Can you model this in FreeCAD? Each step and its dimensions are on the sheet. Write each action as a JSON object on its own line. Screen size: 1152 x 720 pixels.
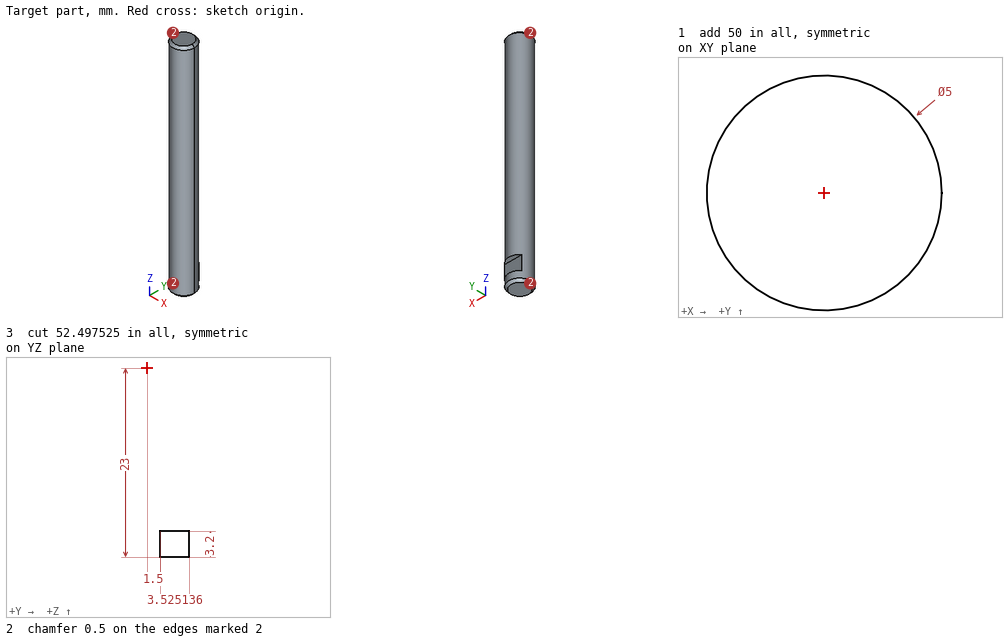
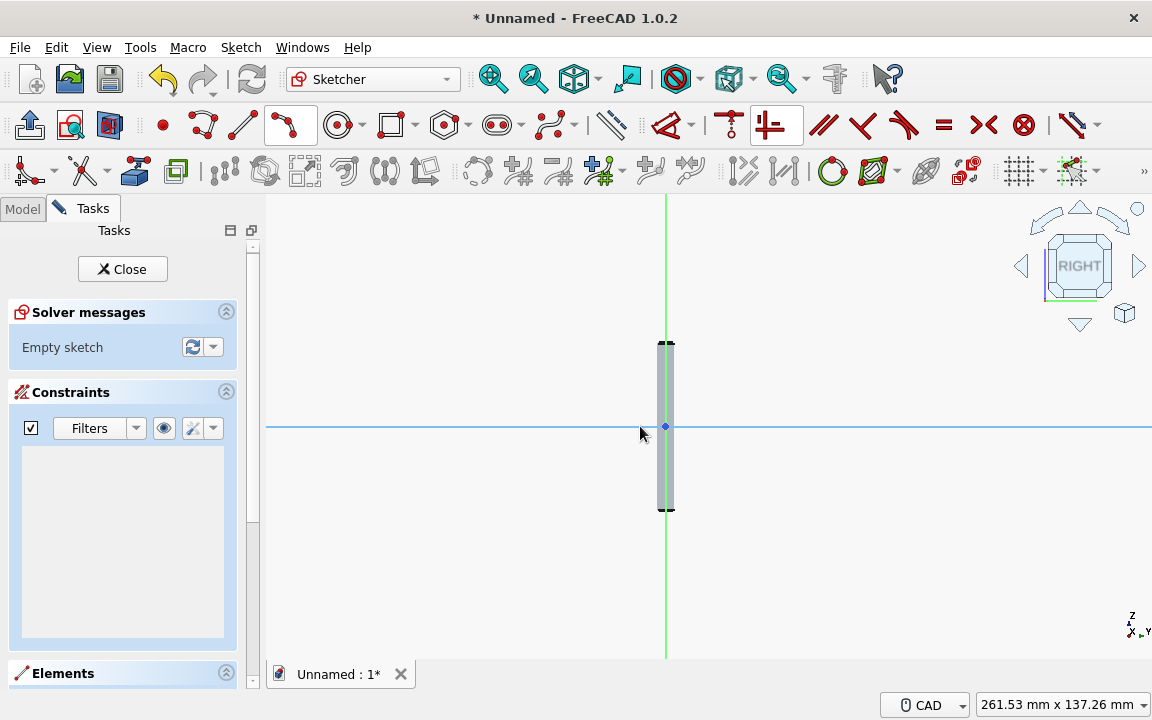
{"action": "scroll", "coordinate": [679, 503], "scroll_direction": "up", "scroll_amount": 15}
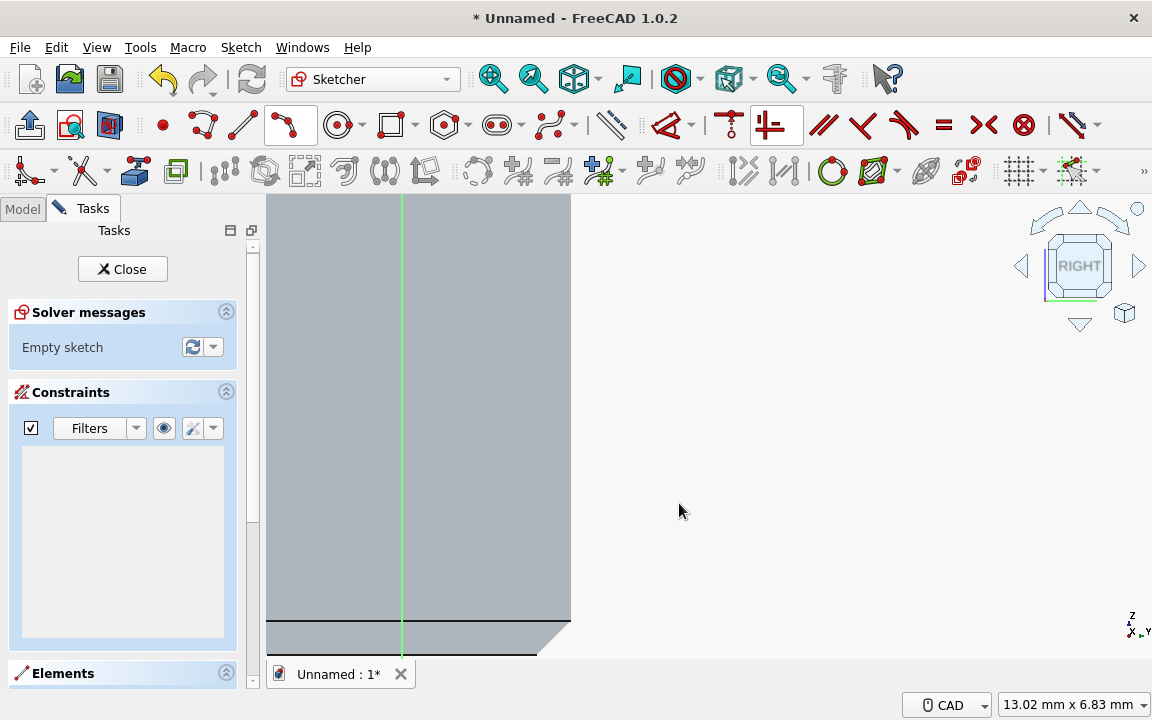
{"action": "key", "text": "g r"}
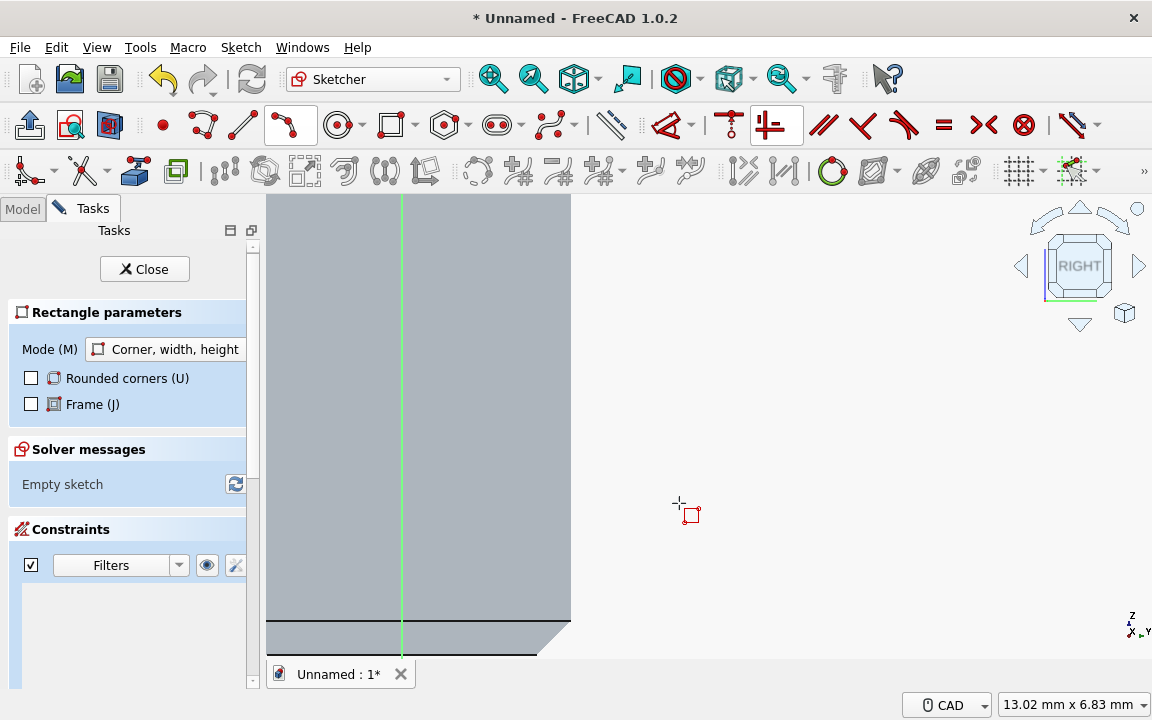
{"action": "left_click", "coordinate": [504, 301]}
{"action": "mouse_move", "coordinate": [744, 519]}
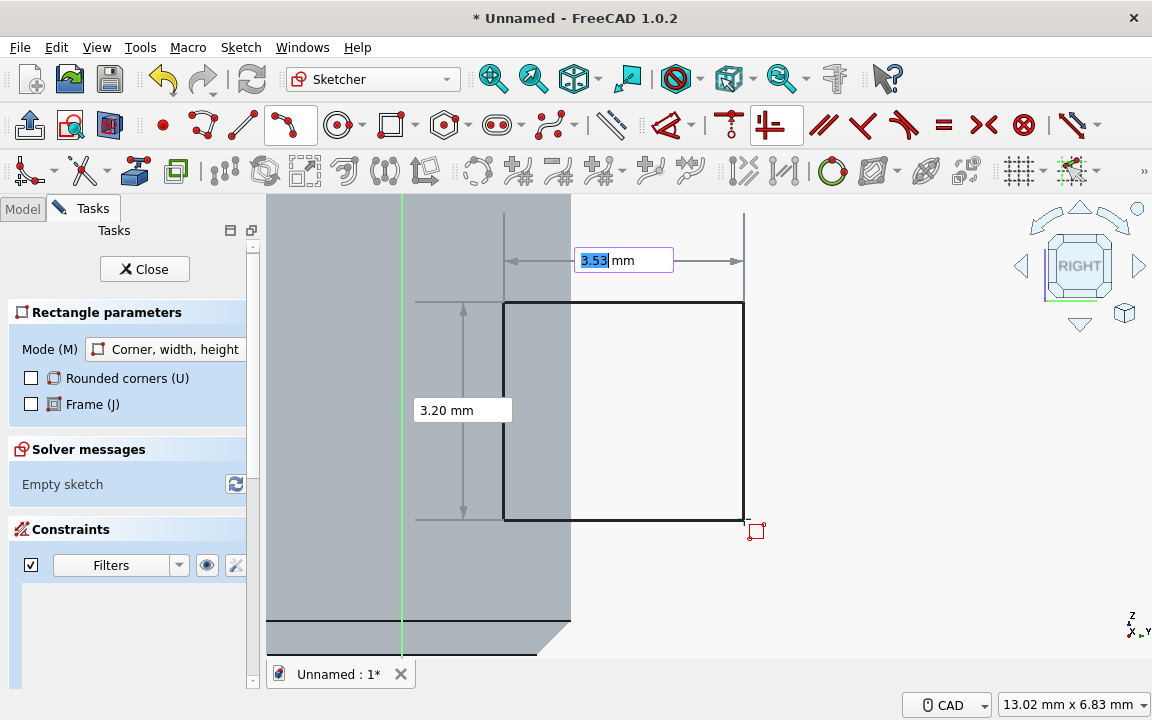
{"action": "type", "text": "3.525136"}
{"action": "key", "text": "Tab"}
{"action": "type", "text": "3.2"}
{"action": "key", "text": "Return"}
{"action": "key", "text": "Escape"}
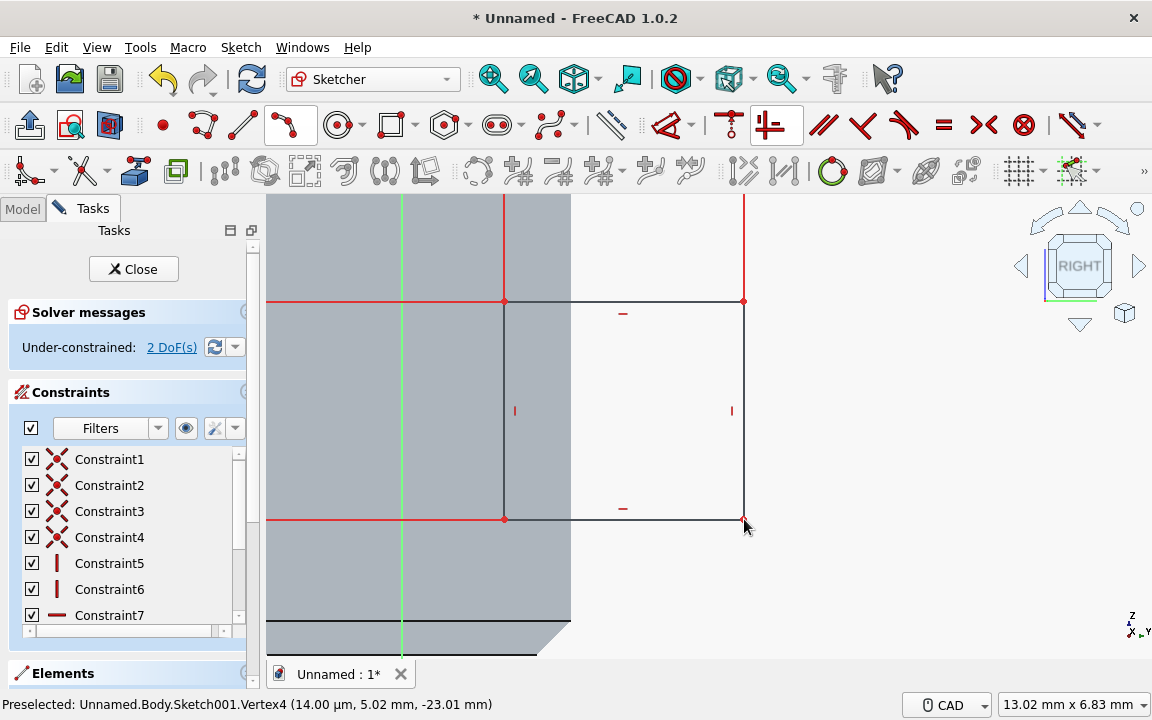
{"action": "left_click", "coordinate": [504, 520]}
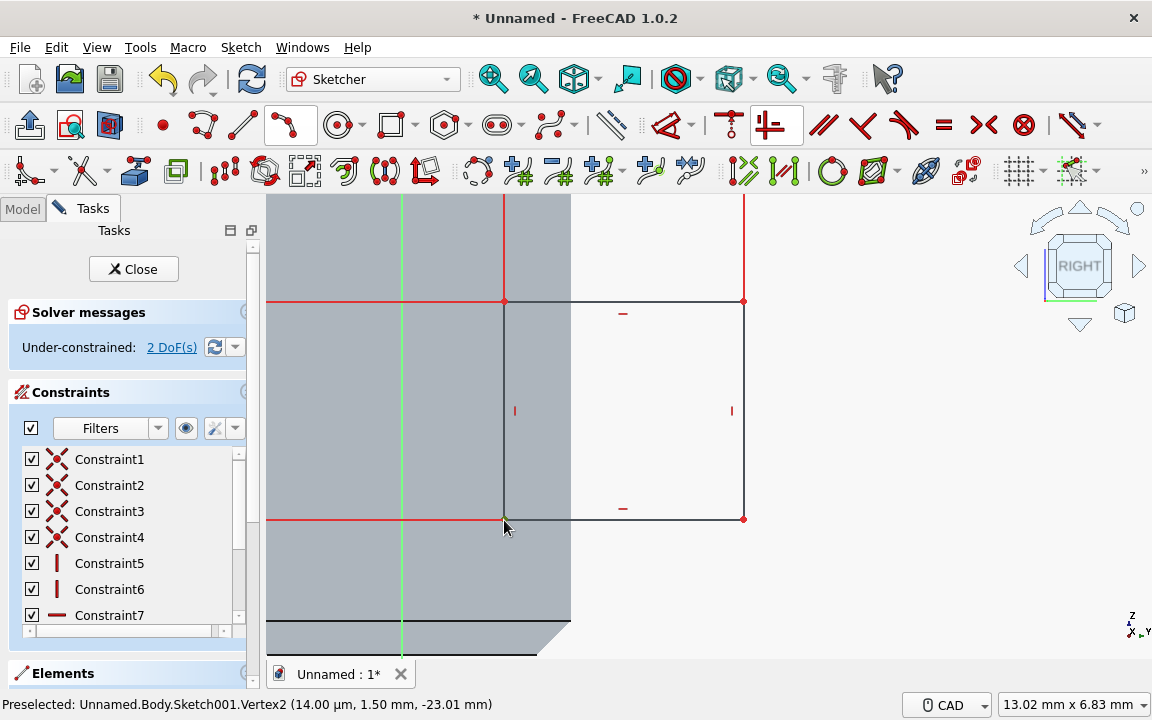
{"action": "key", "text": "i"}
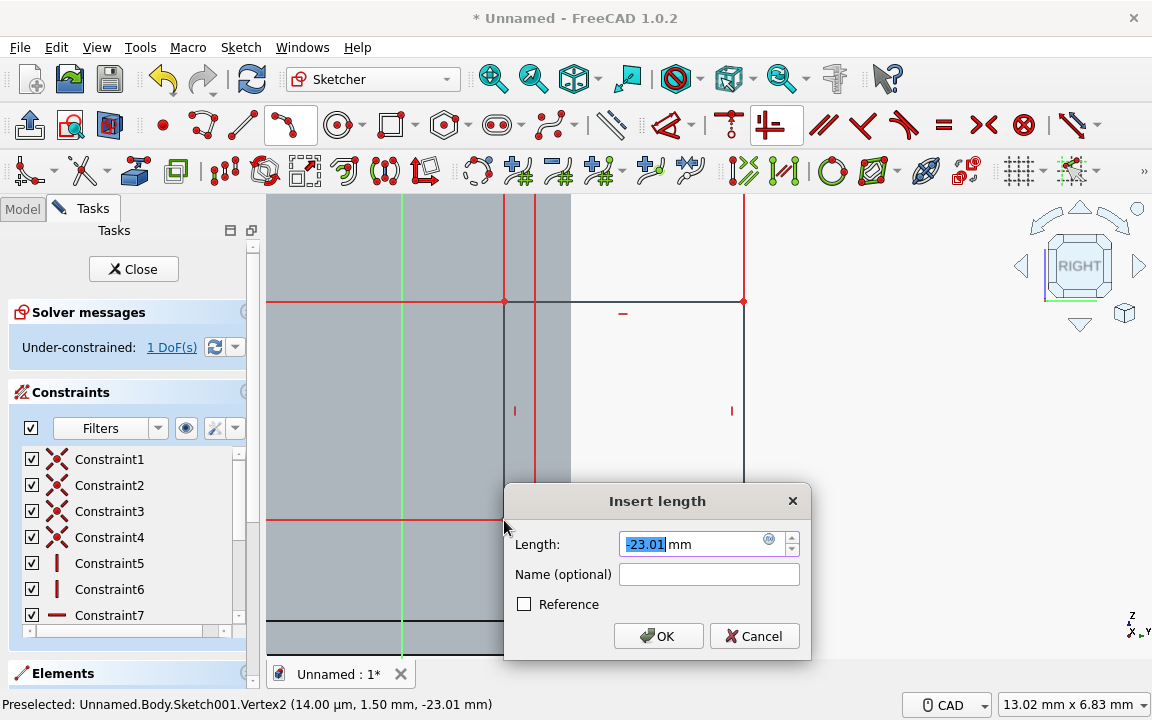
{"action": "type", "text": "-23"}
{"action": "key", "text": "Return"}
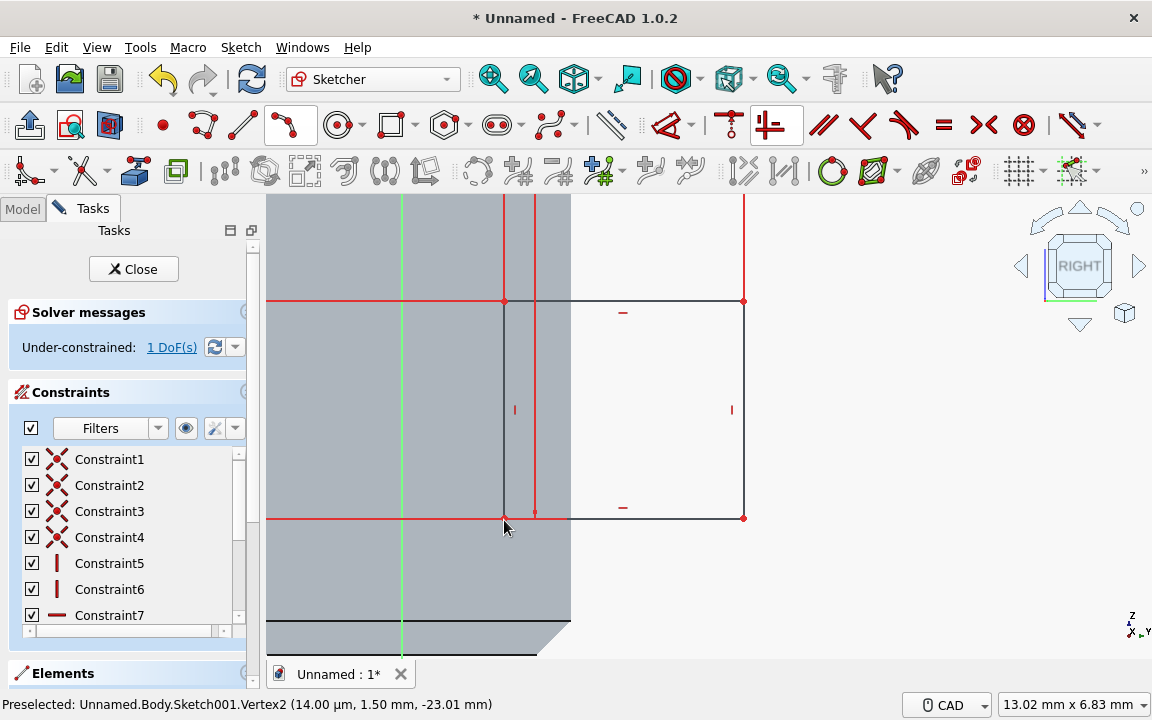
{"action": "left_click", "coordinate": [504, 301]}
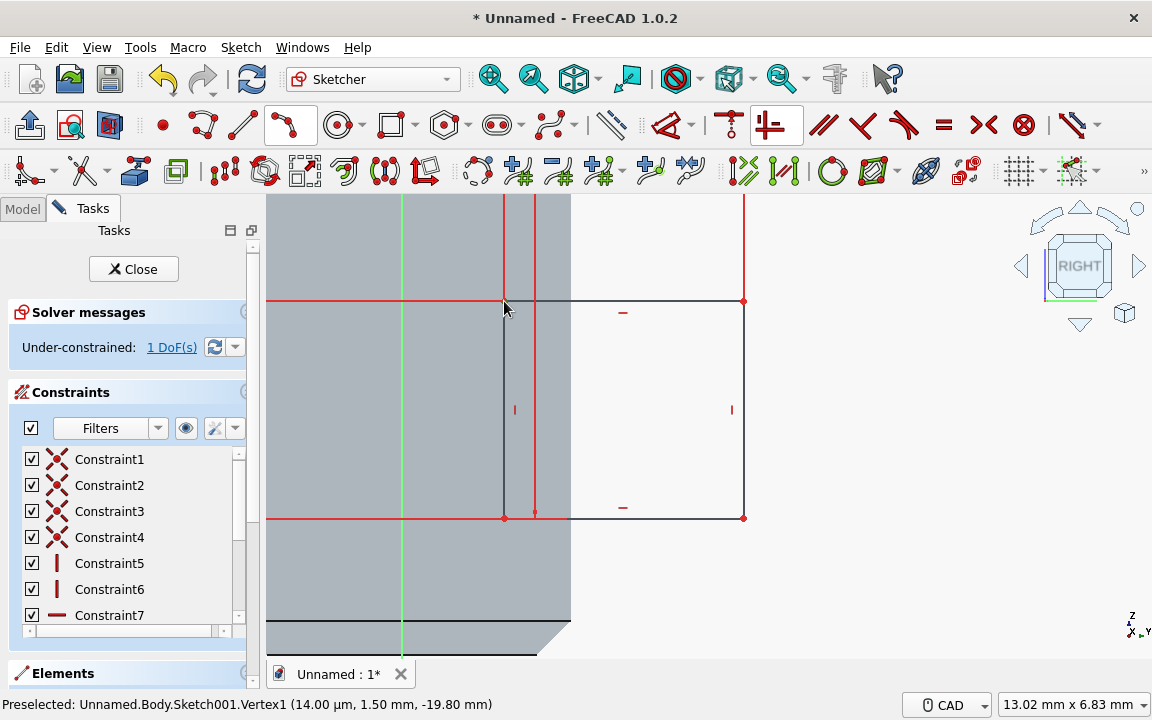
{"action": "key", "text": "l"}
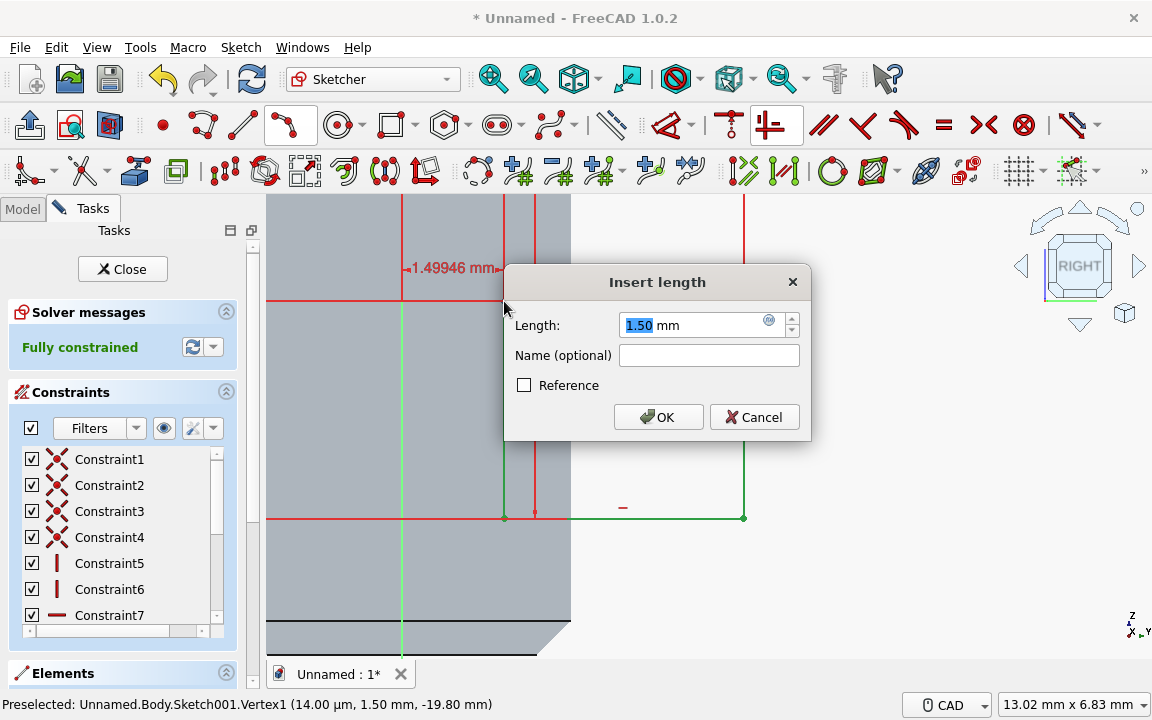
{"action": "type", "text": "1.5"}
{"action": "key", "text": "Return"}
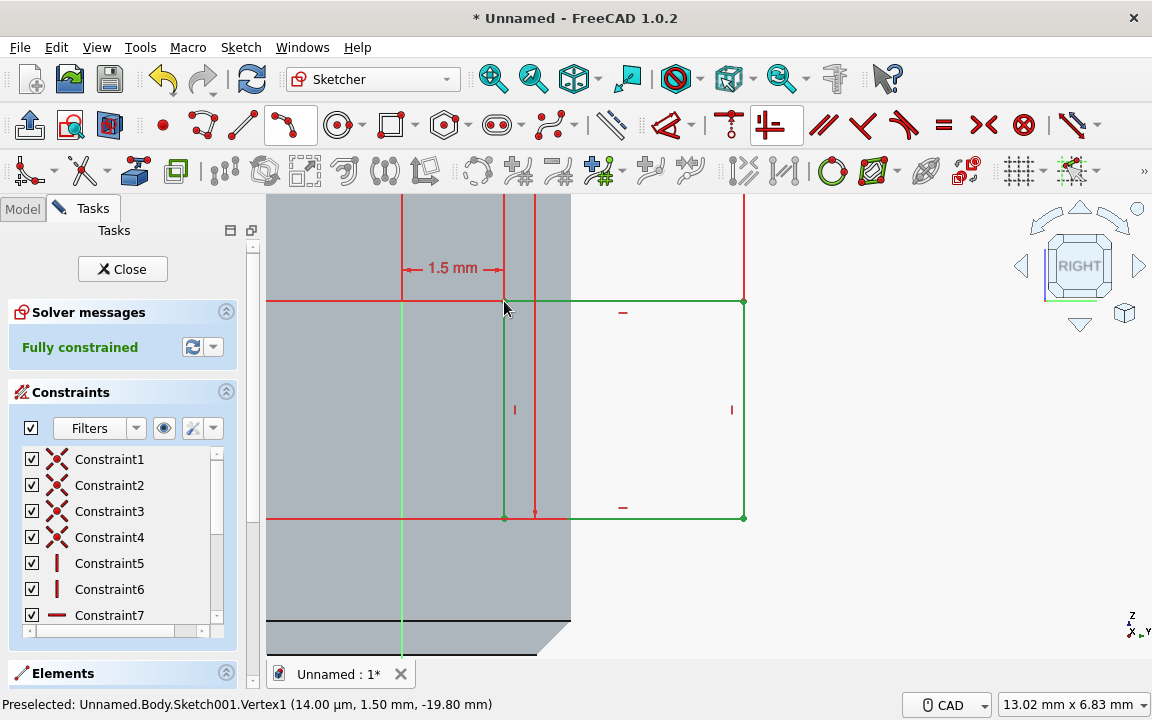
{"action": "left_click", "coordinate": [123, 269]}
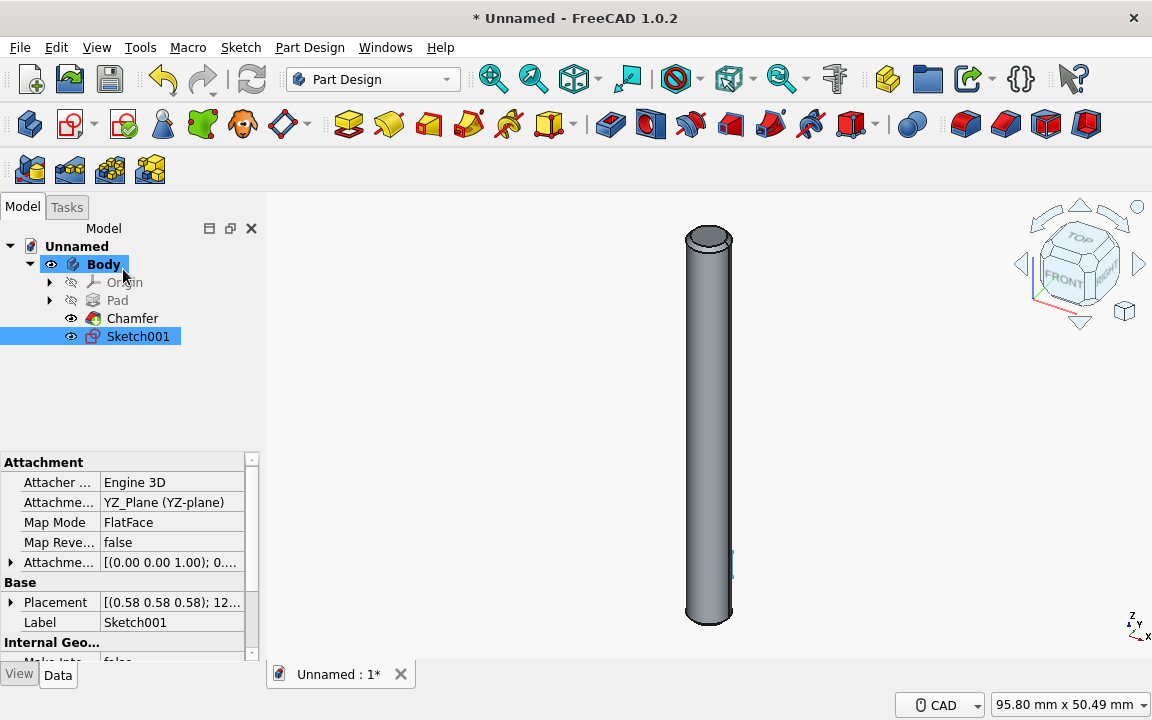
{"action": "left_click", "coordinate": [612, 124]}